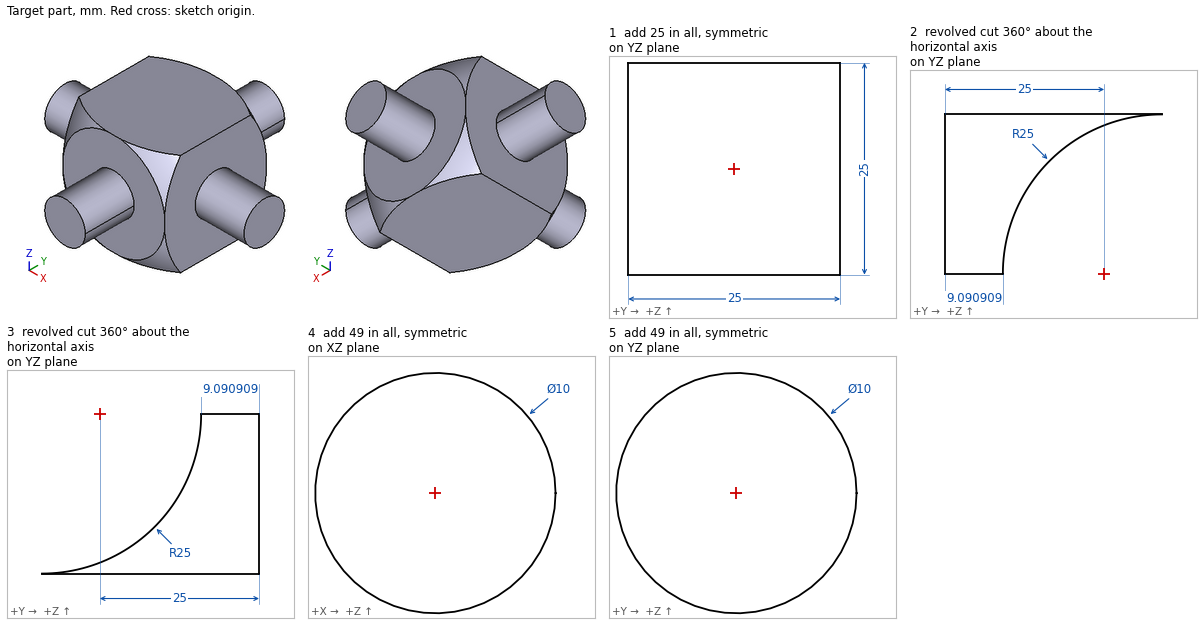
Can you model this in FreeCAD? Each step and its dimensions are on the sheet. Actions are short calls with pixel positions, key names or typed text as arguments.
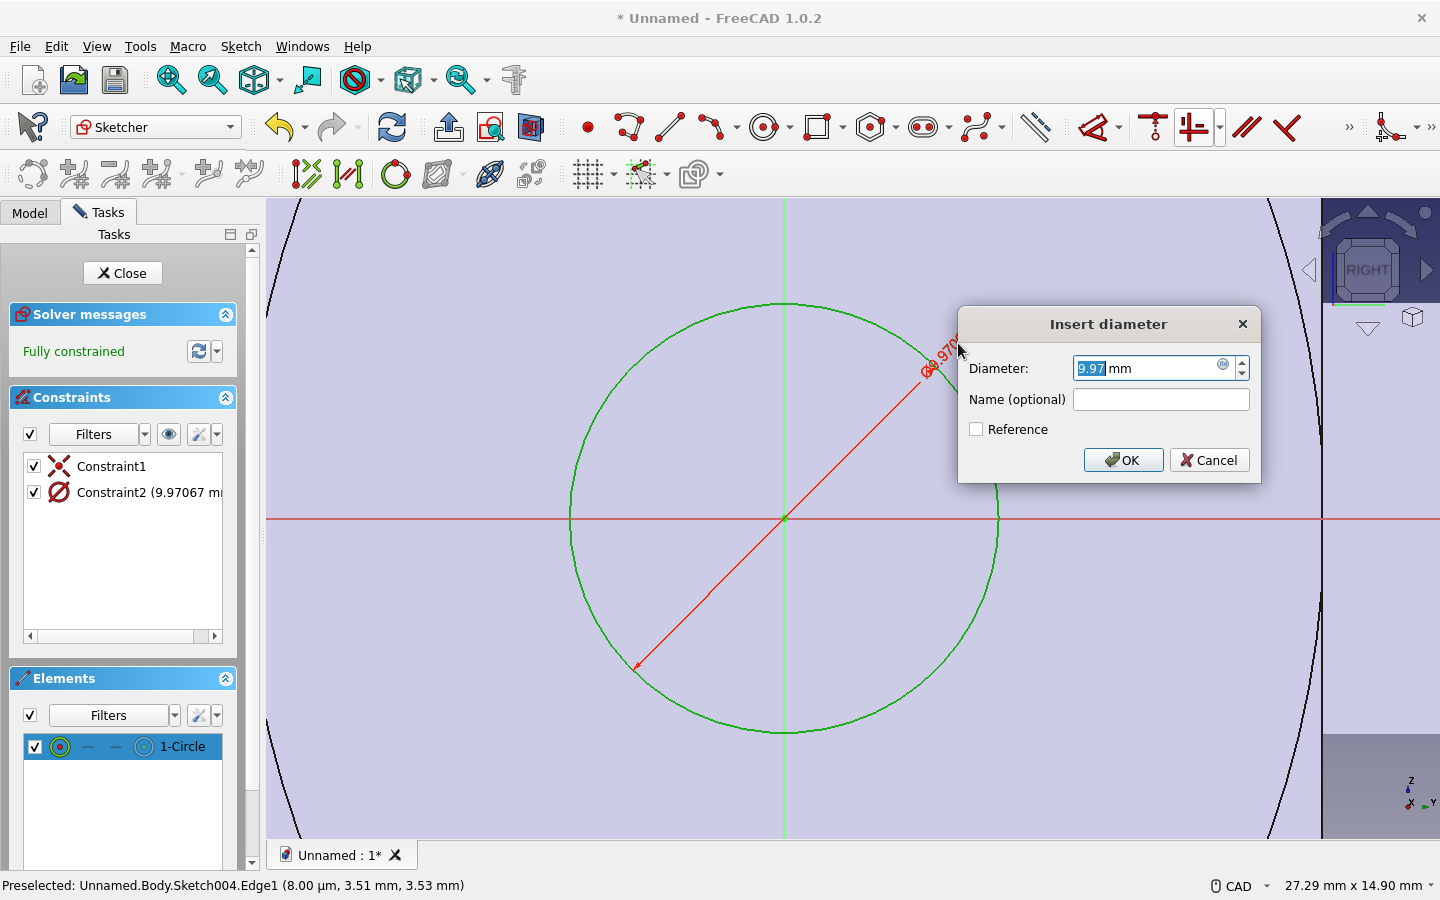
text(10)
key(Return)
key(Escape)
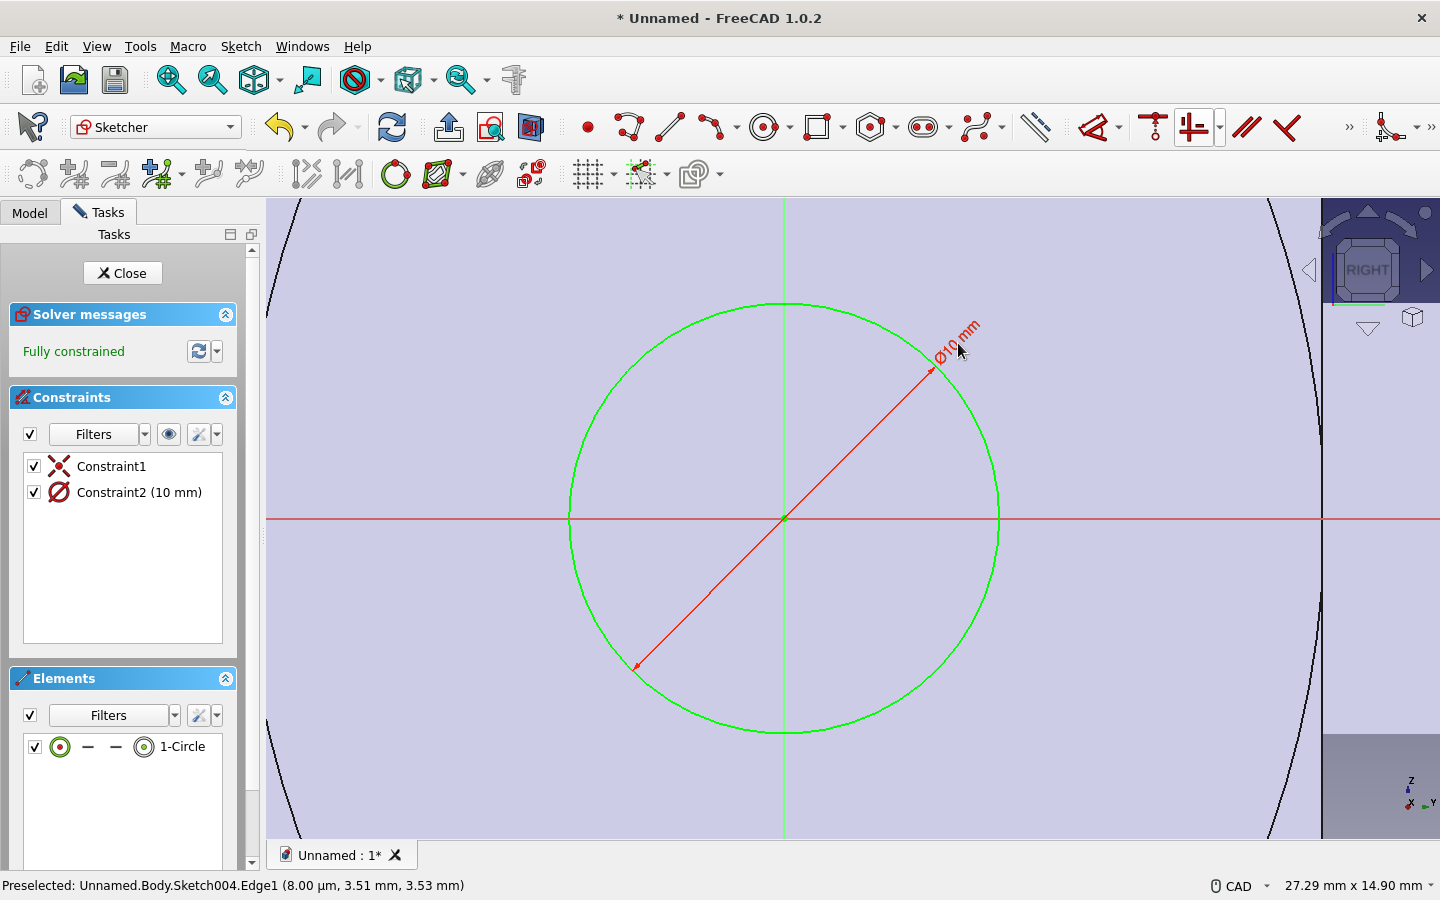
click(123, 273)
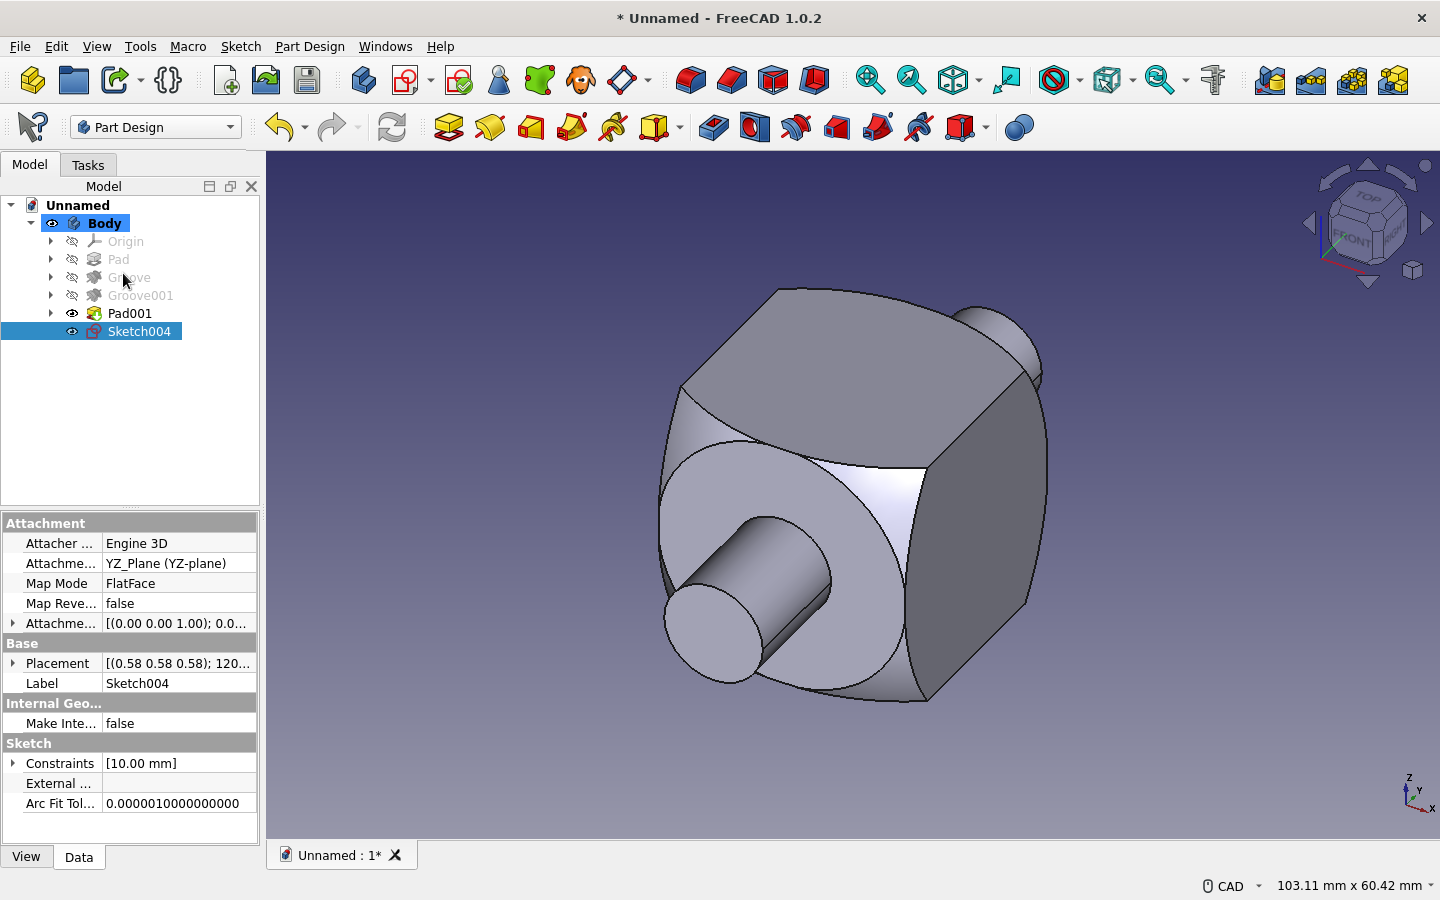
click(449, 128)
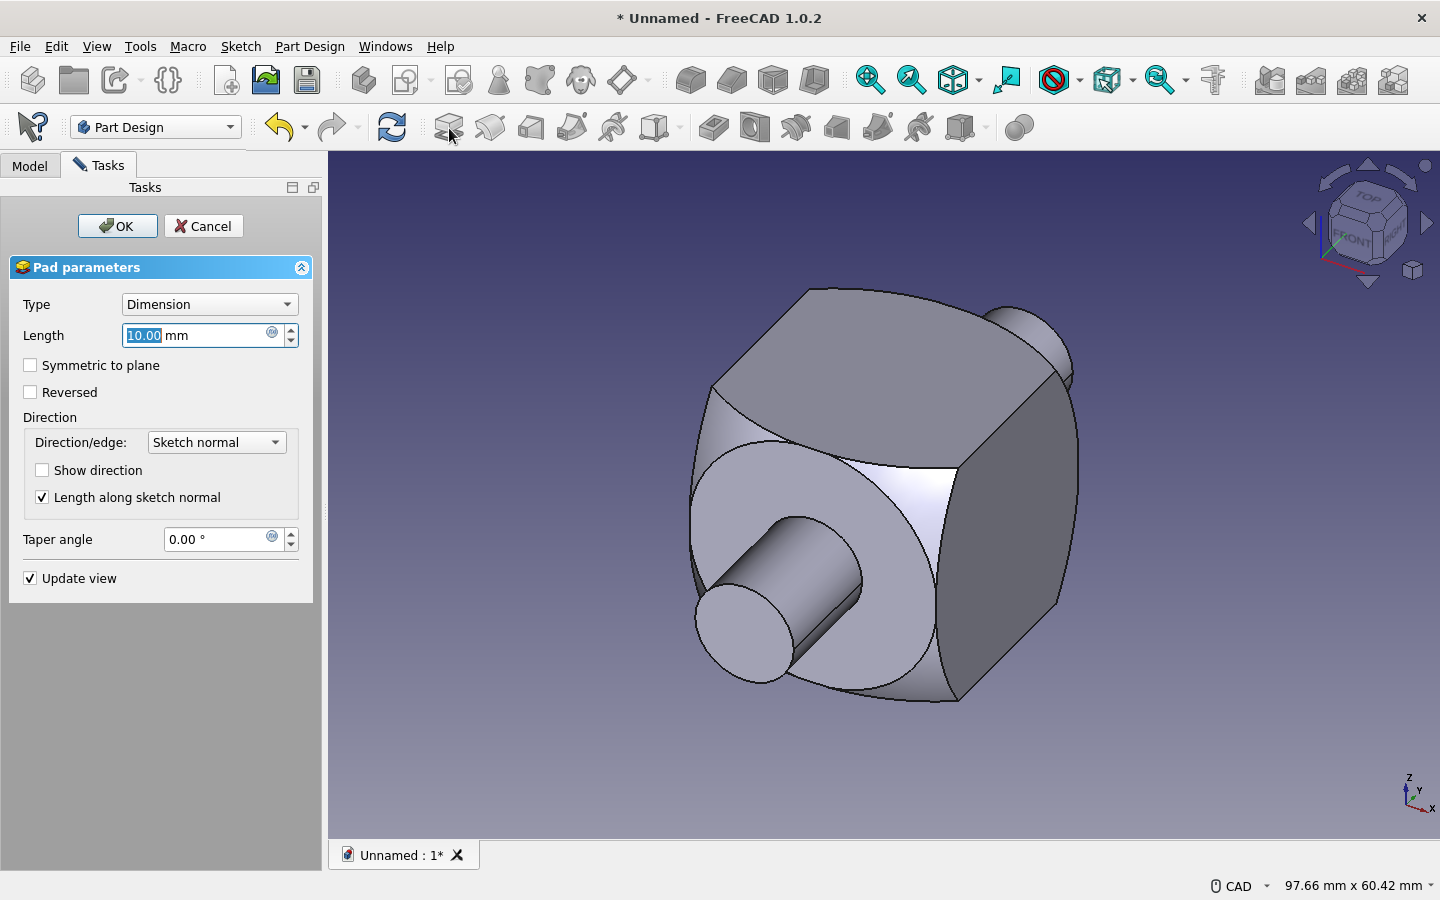
text(49)
key(Tab)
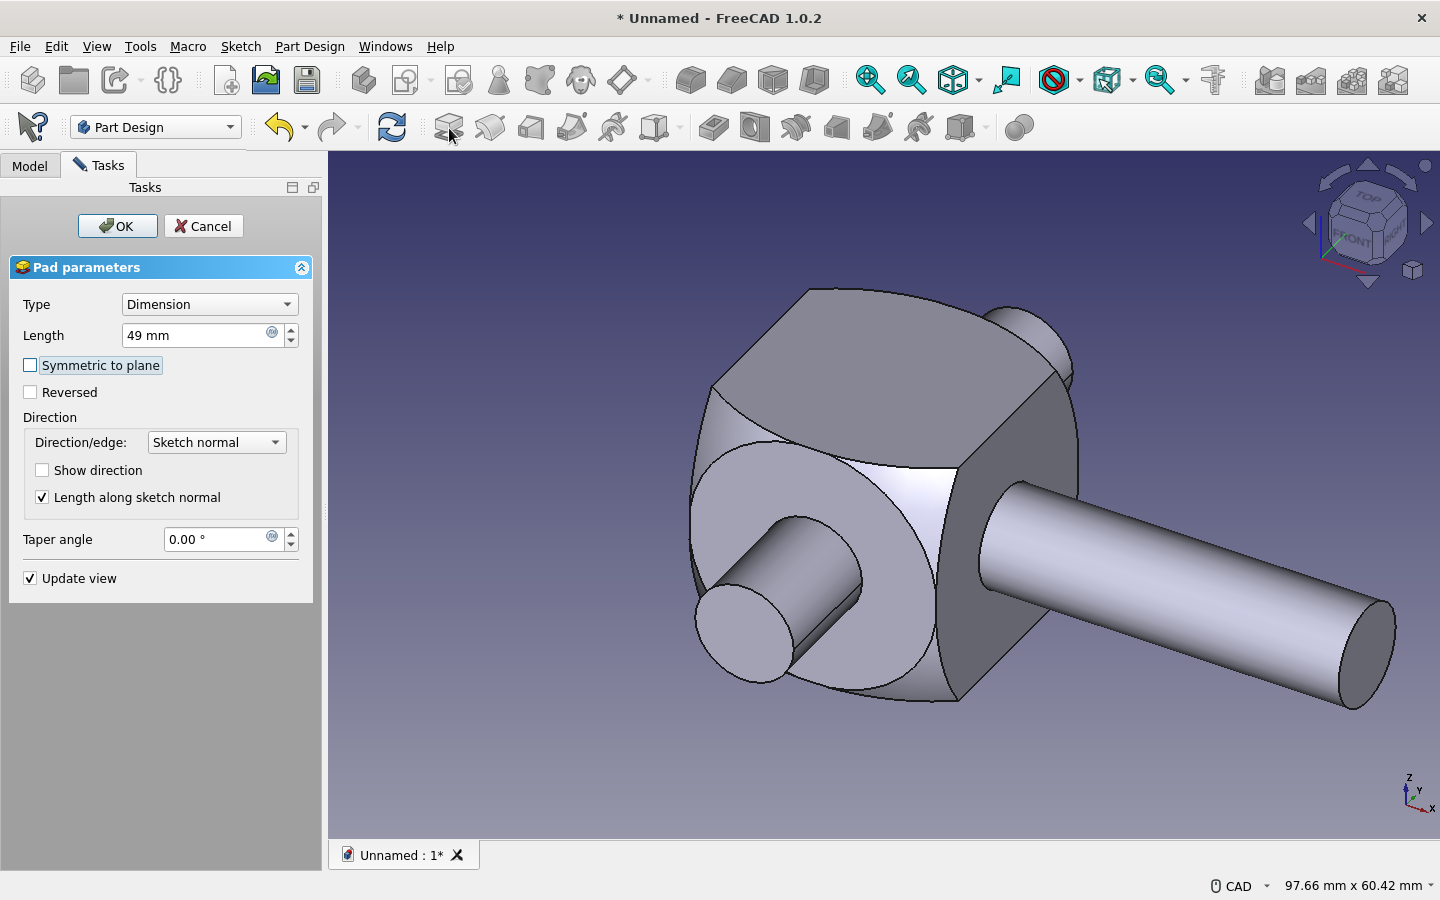
click(31, 365)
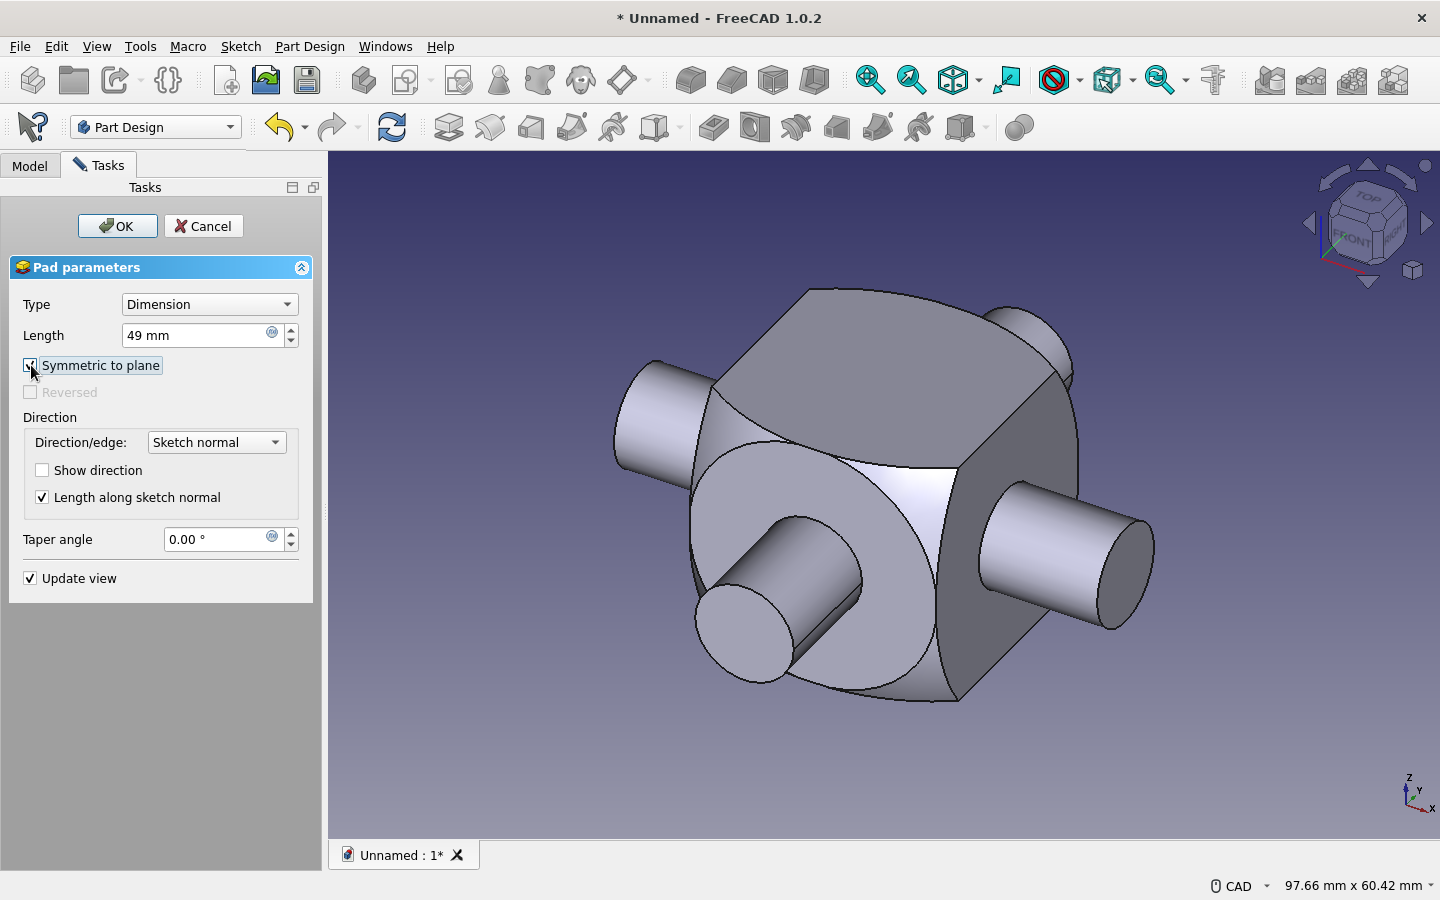
click(118, 226)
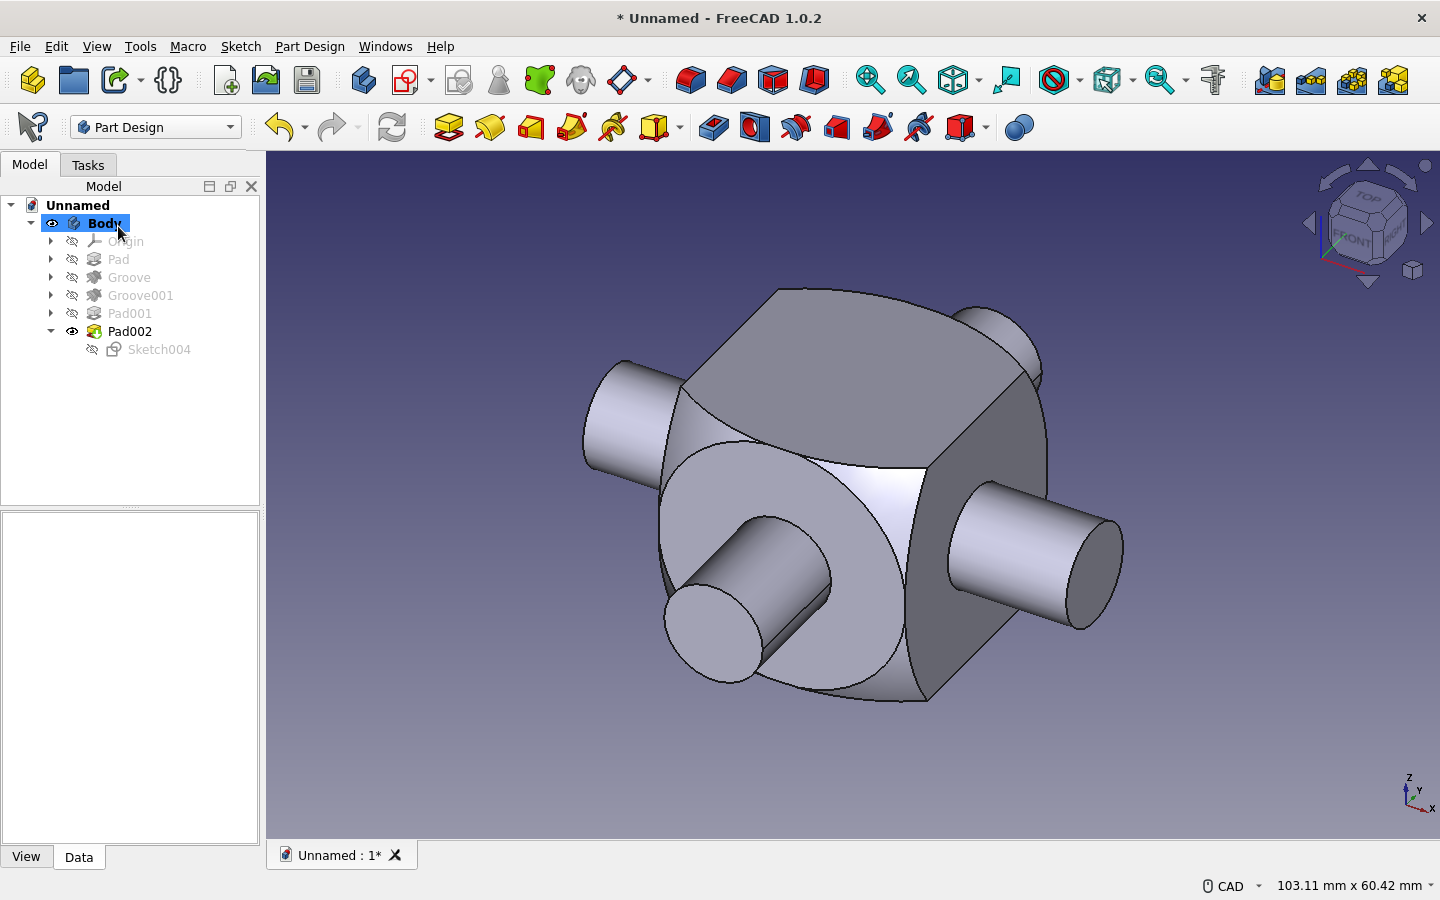
key(0)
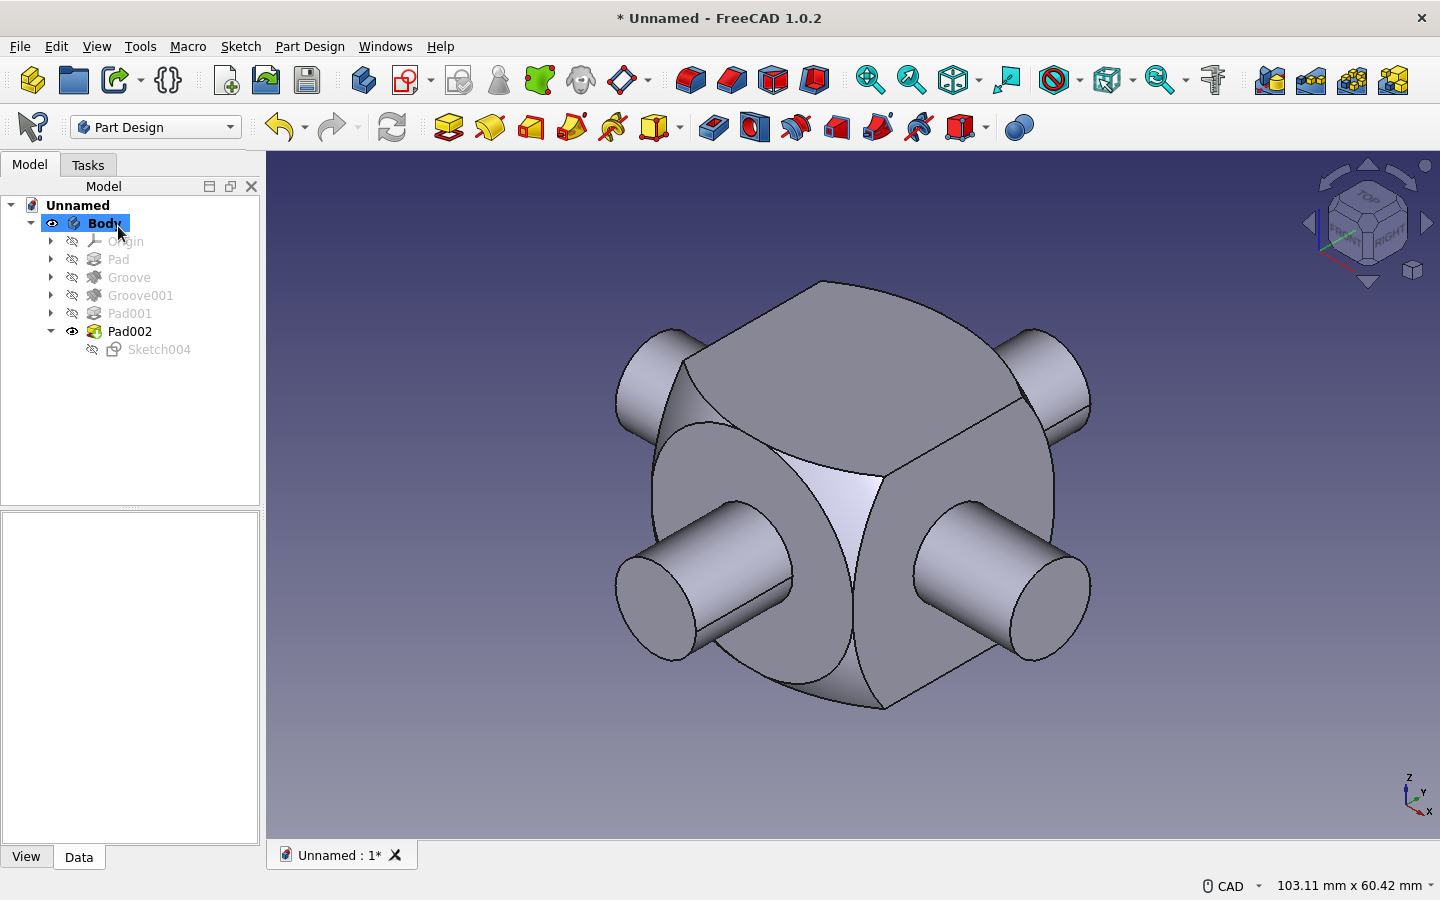
click(871, 80)